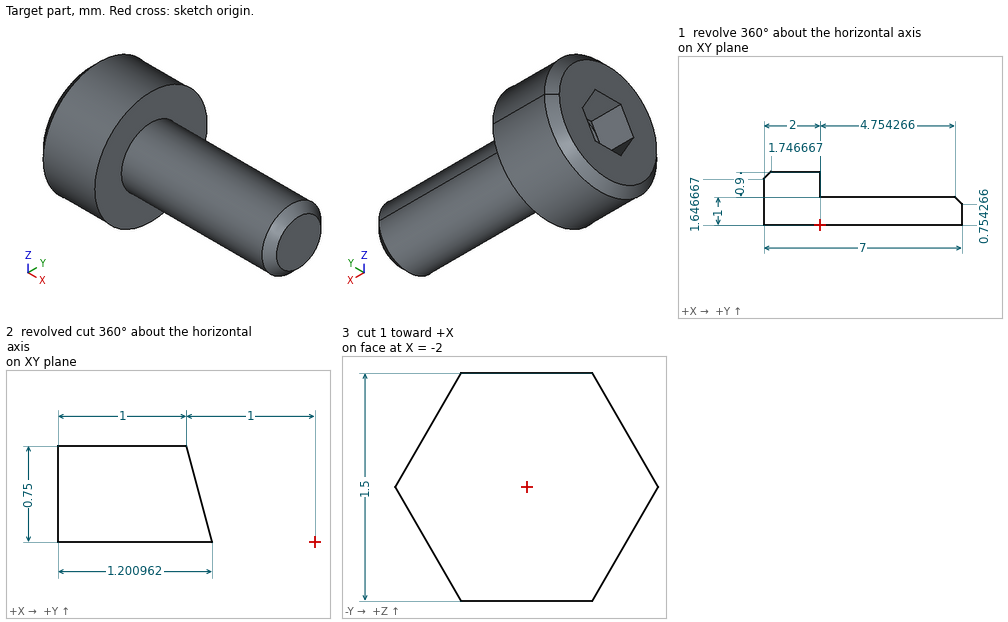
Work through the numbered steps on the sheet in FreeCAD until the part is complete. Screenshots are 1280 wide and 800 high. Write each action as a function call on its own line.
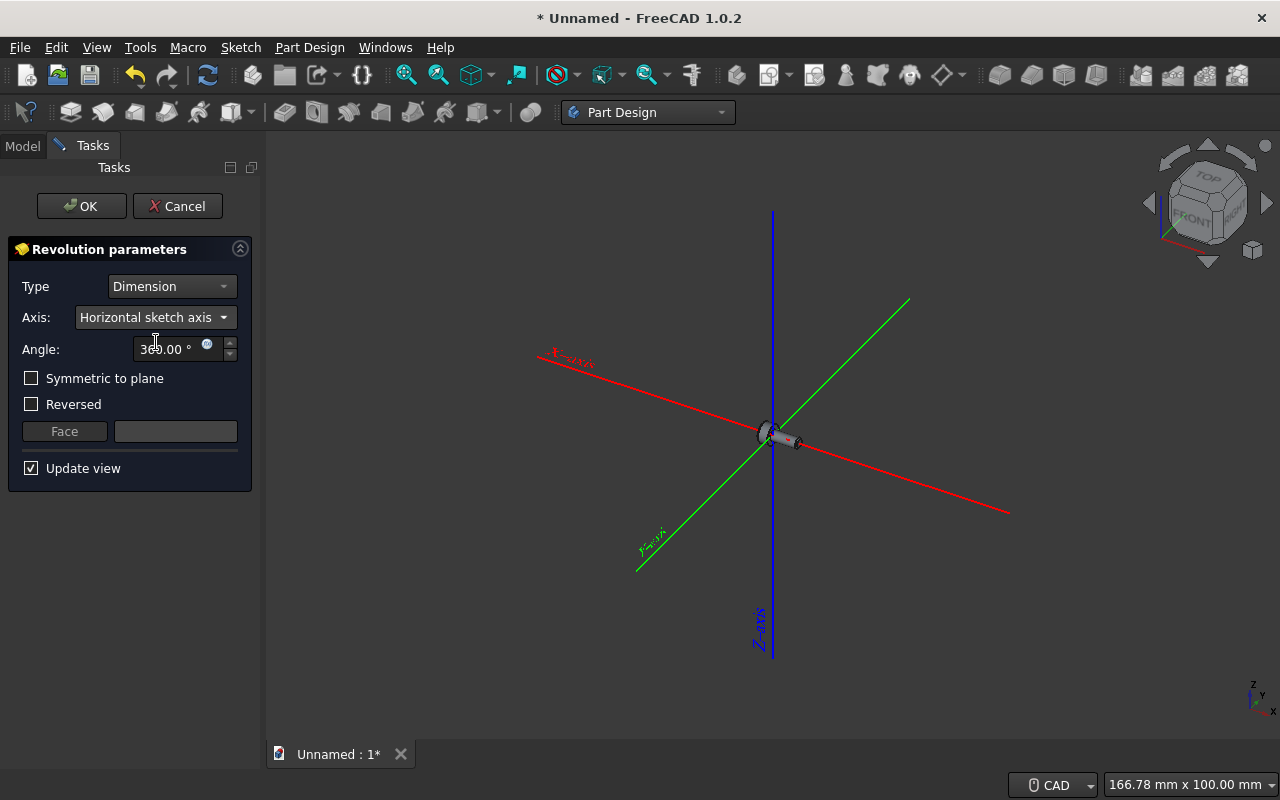
click(82, 206)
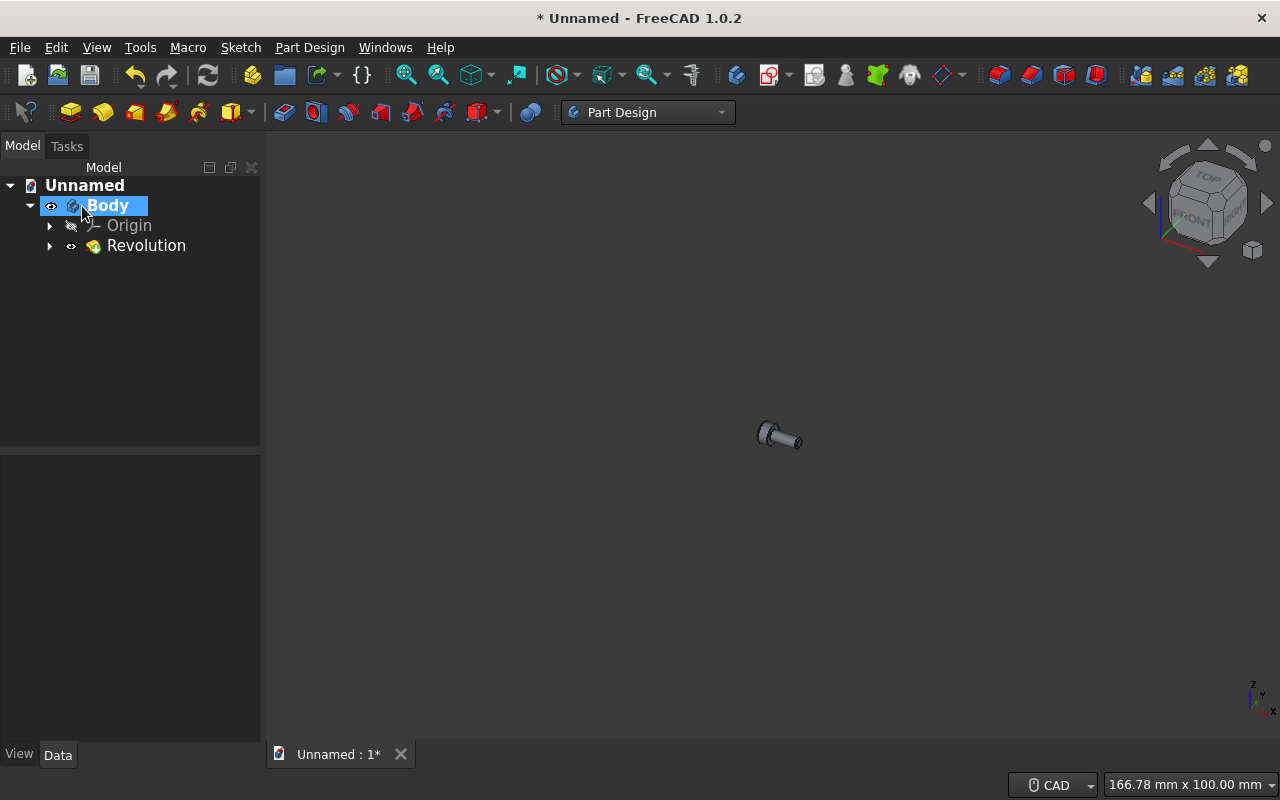
click(408, 76)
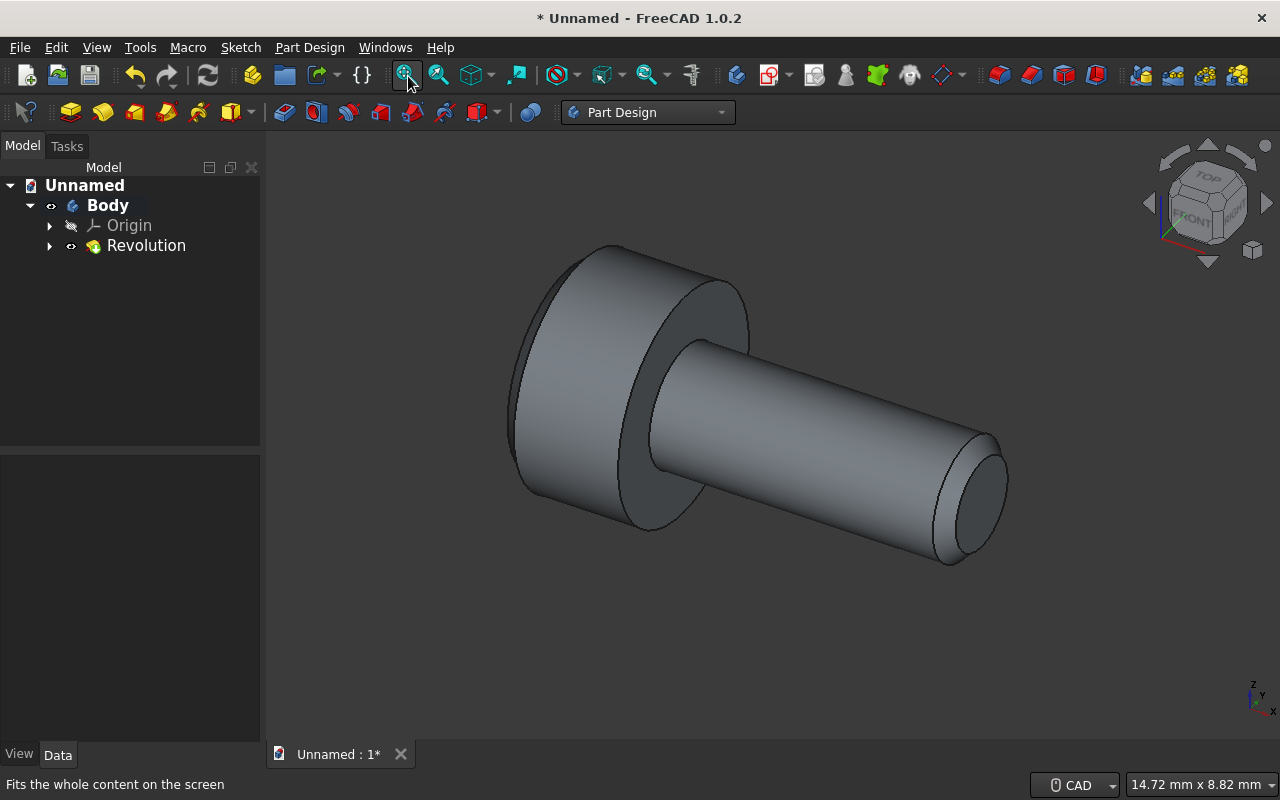
click(770, 76)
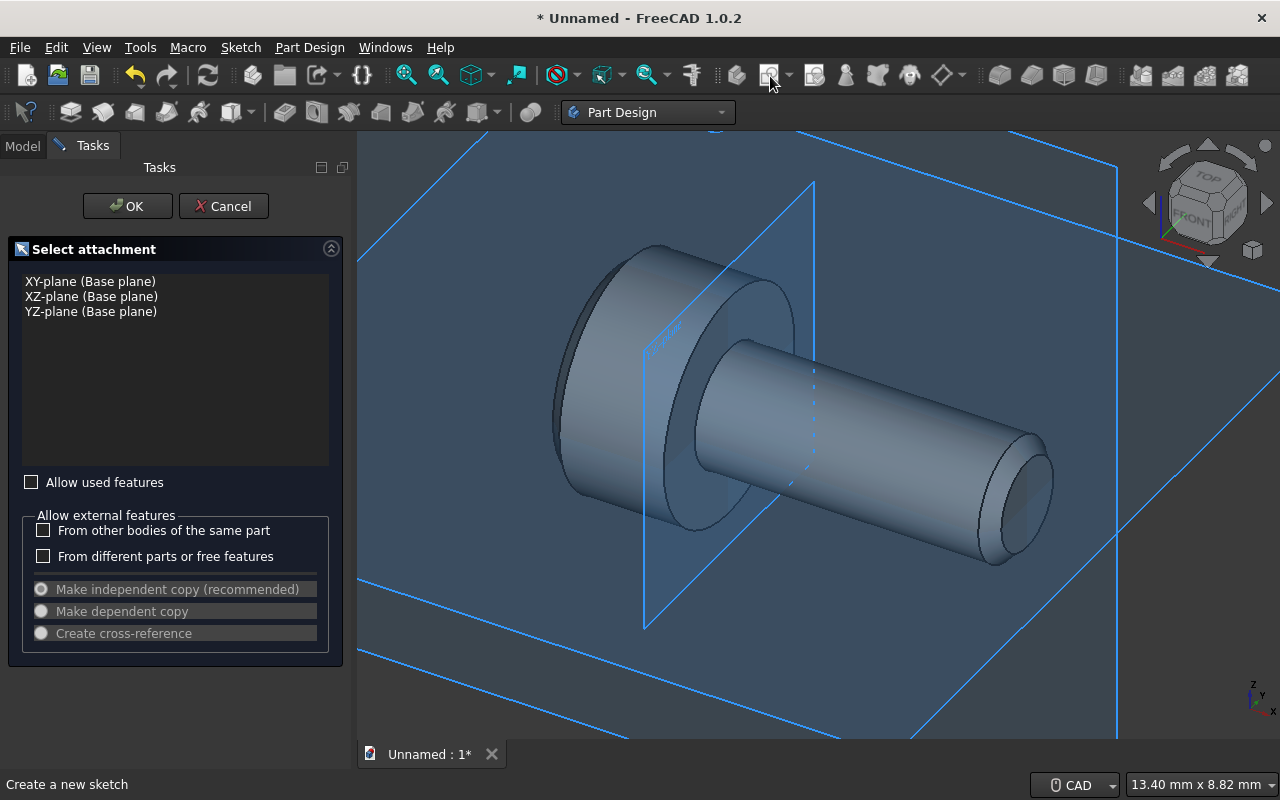
click(82, 282)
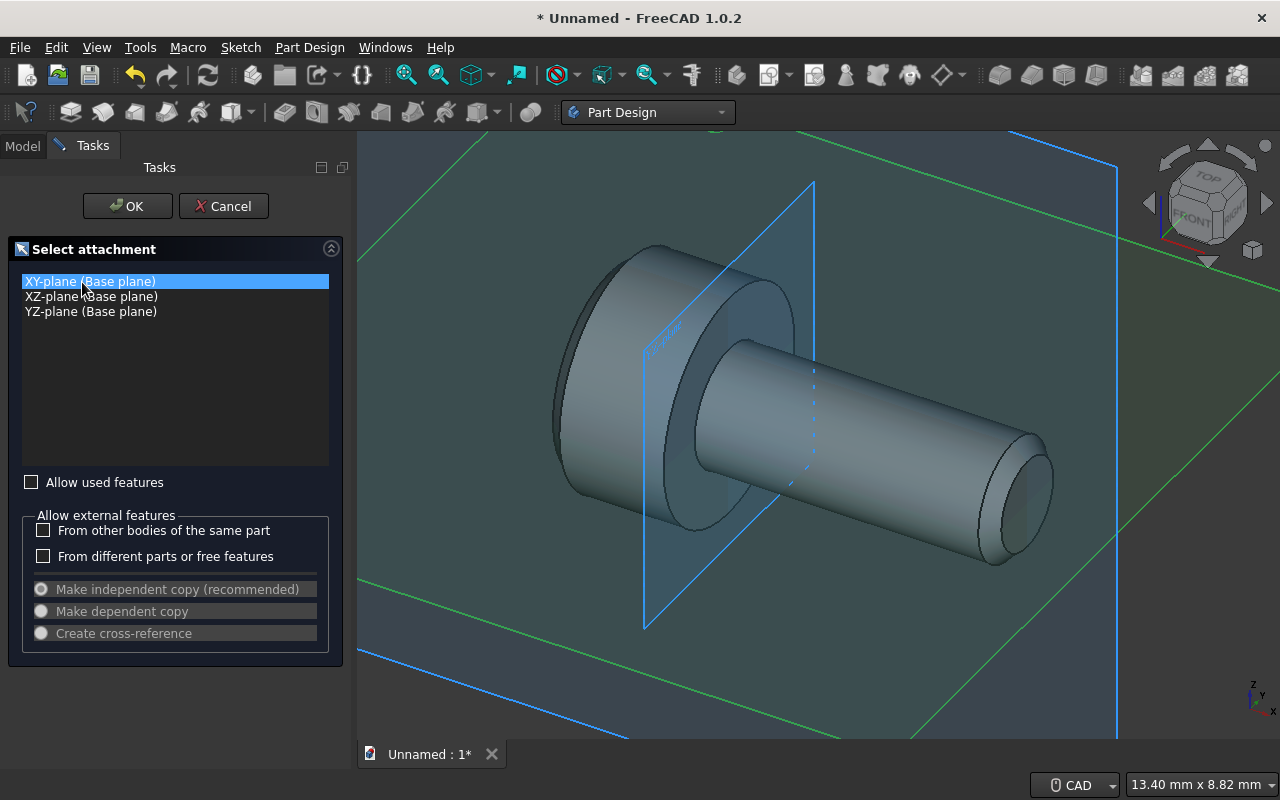
click(128, 206)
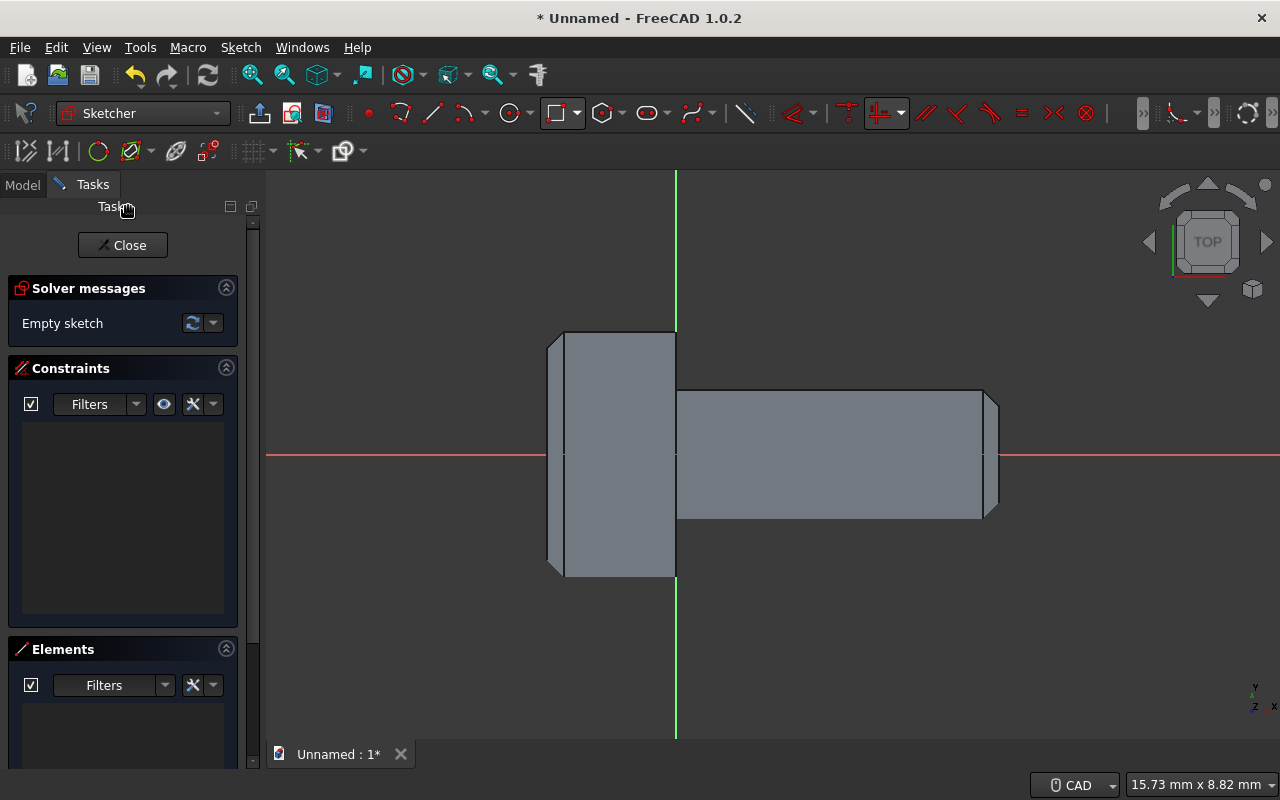
click(324, 114)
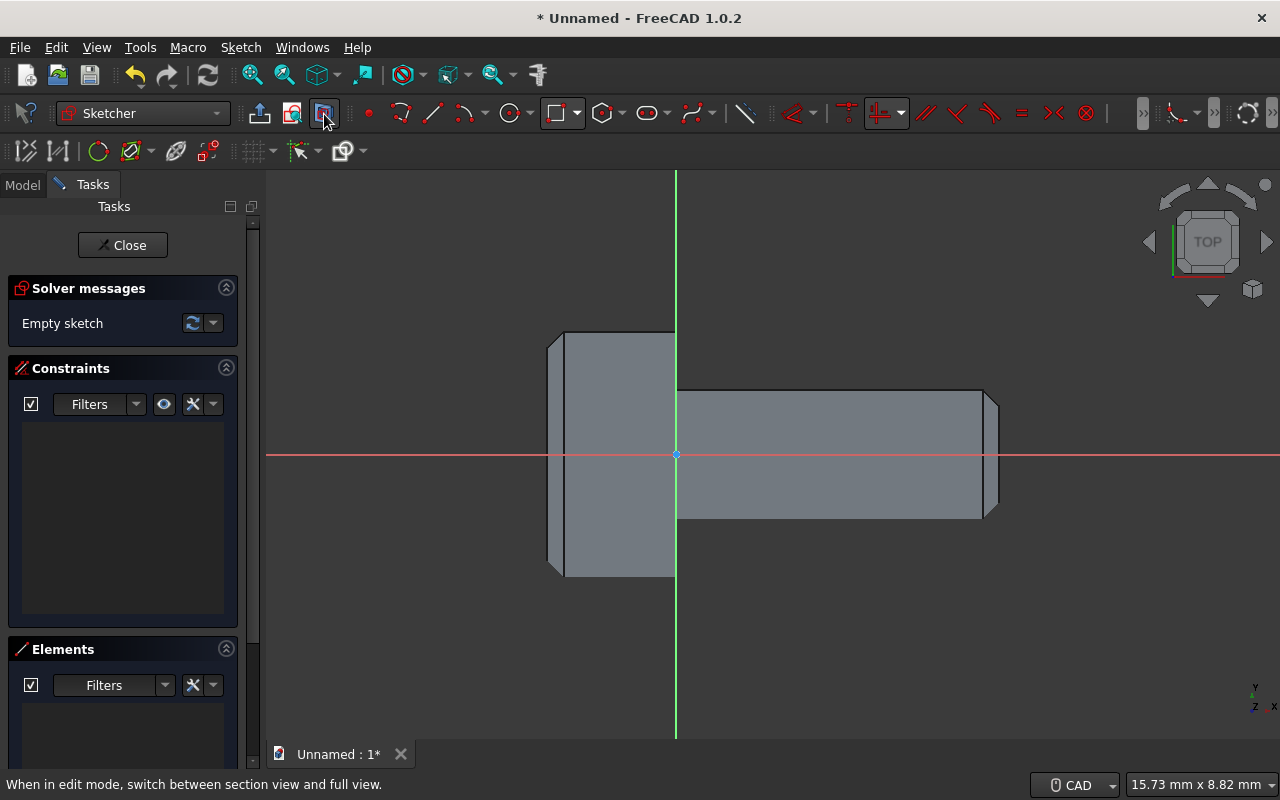
scroll(588, 424, up, 8)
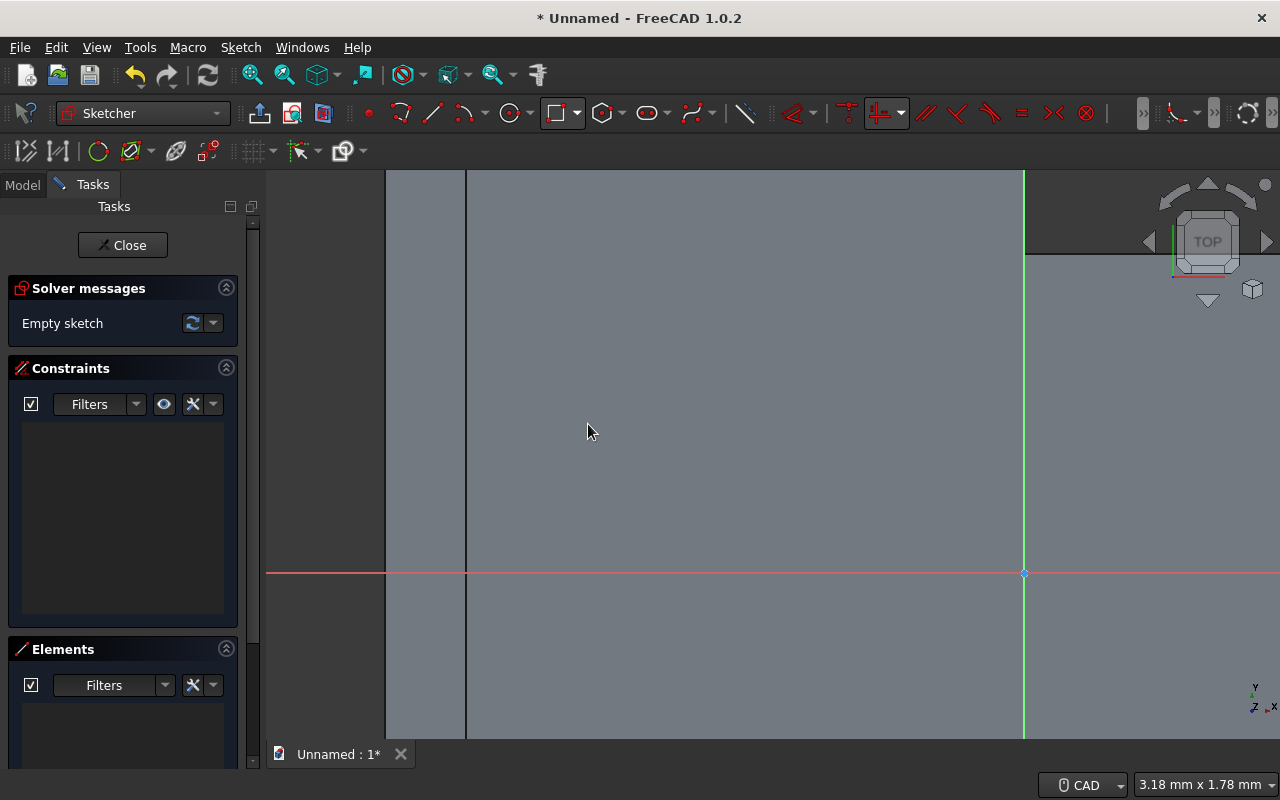
click(402, 114)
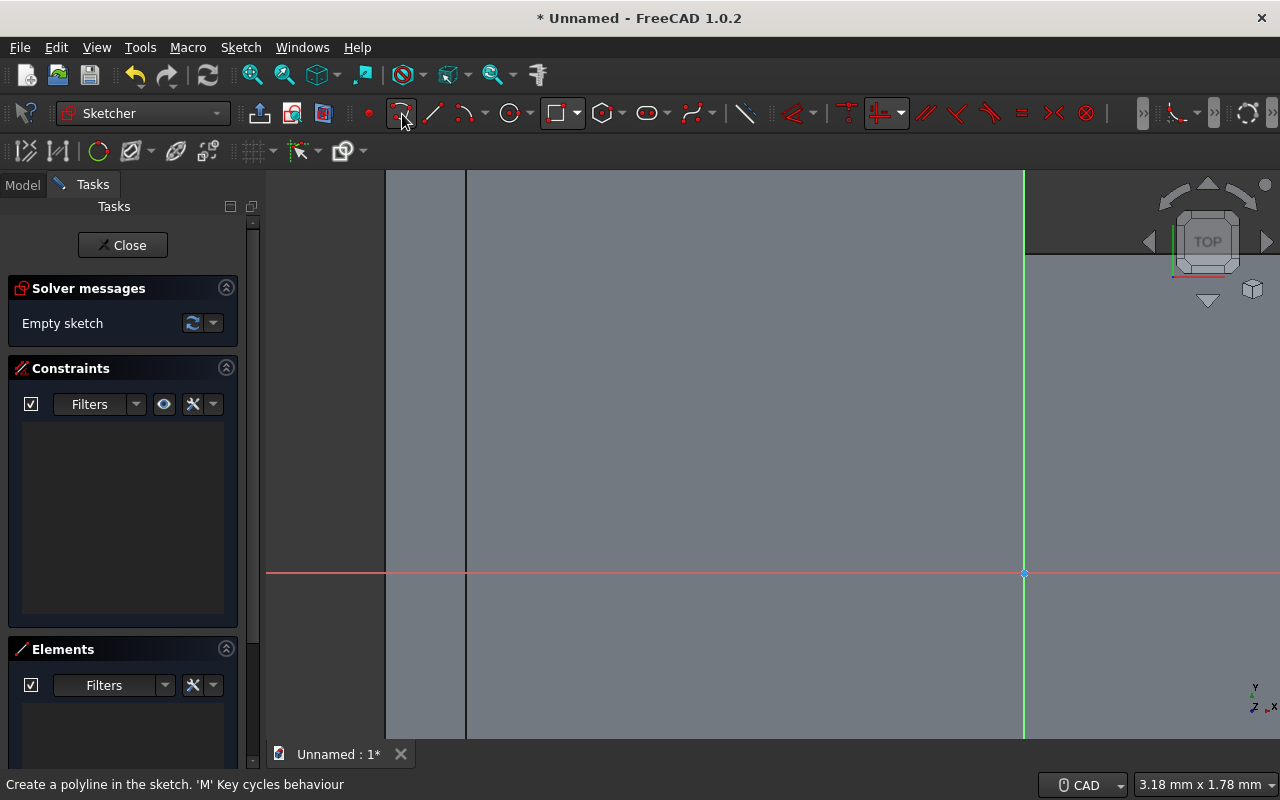
click(769, 573)
click(705, 334)
click(385, 334)
click(385, 564)
click(769, 573)
key(Escape)
key(Escape)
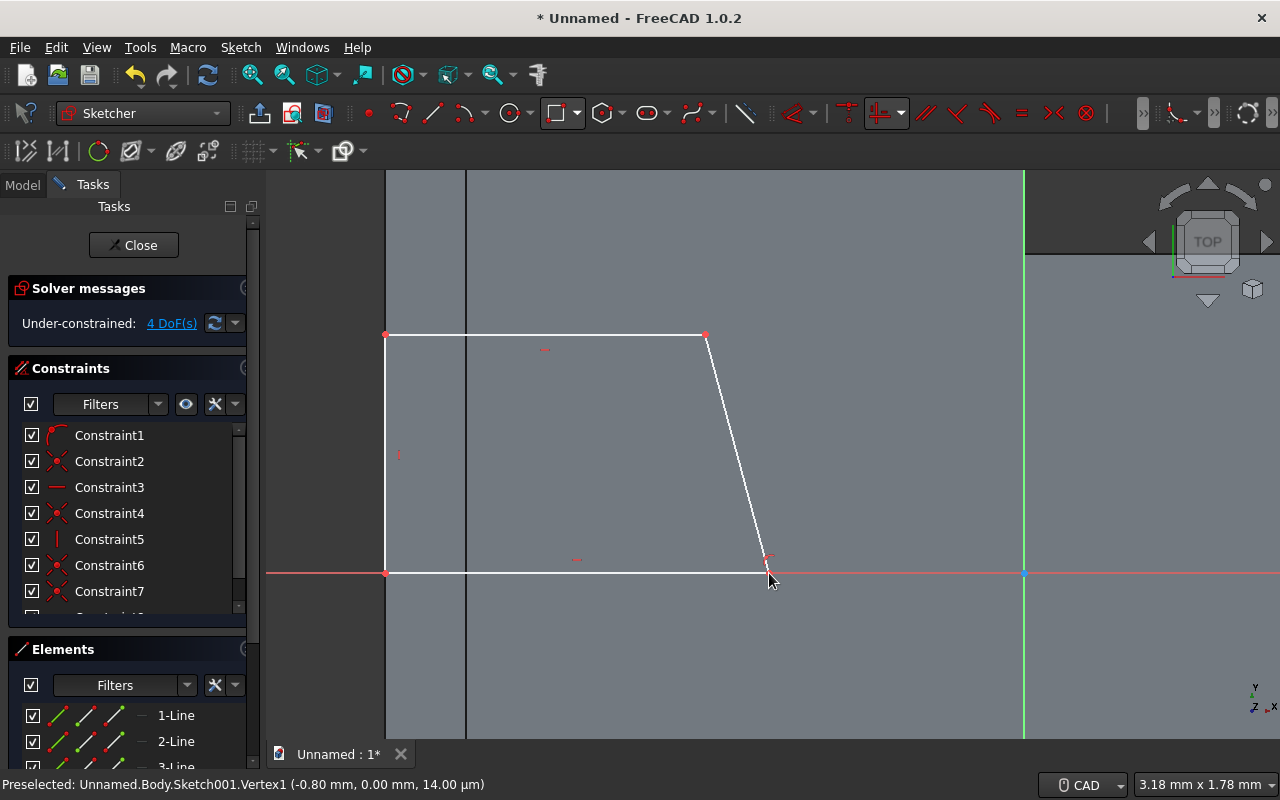
click(792, 114)